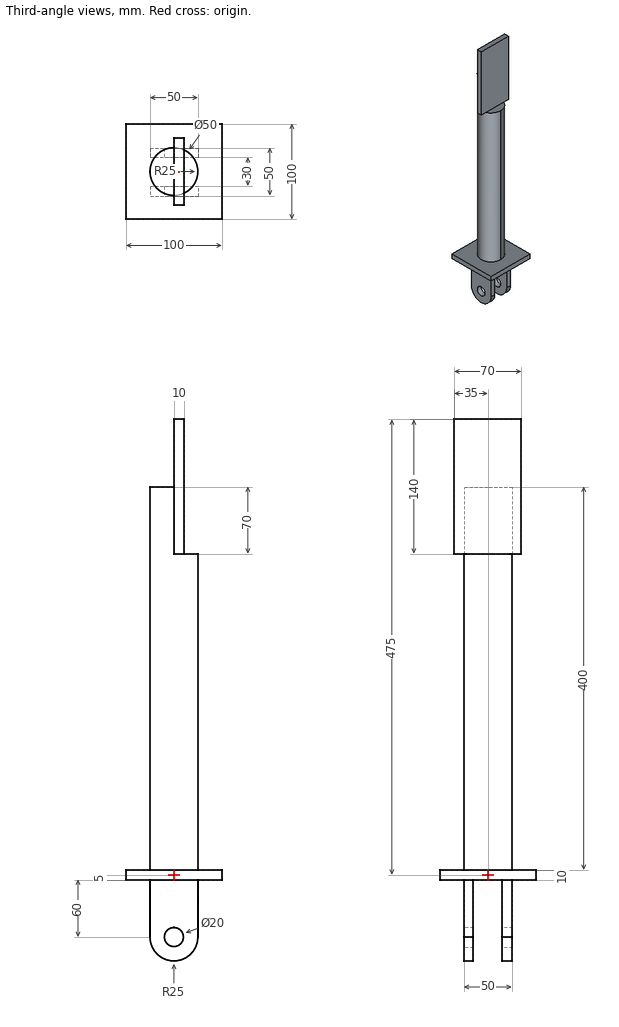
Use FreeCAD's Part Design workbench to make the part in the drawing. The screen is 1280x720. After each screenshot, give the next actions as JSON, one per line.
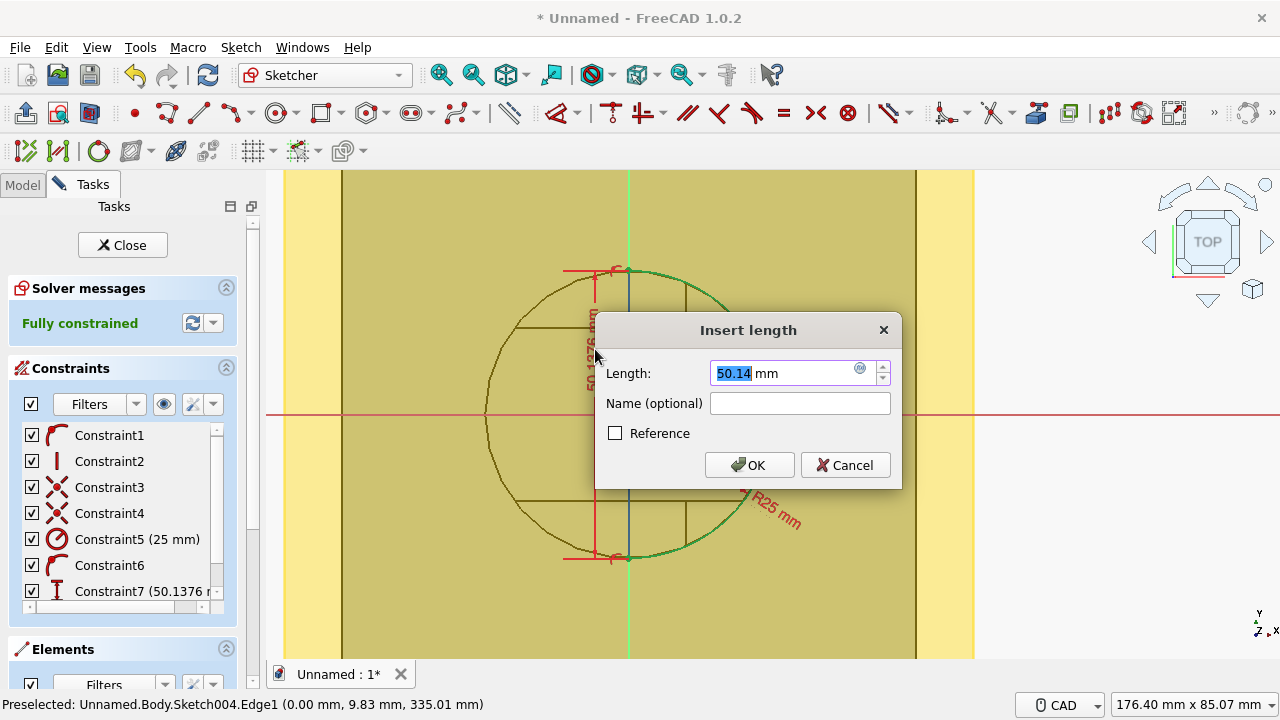
{"action": "type", "text": "50"}
{"action": "key", "text": "Return"}
{"action": "key", "text": "Escape"}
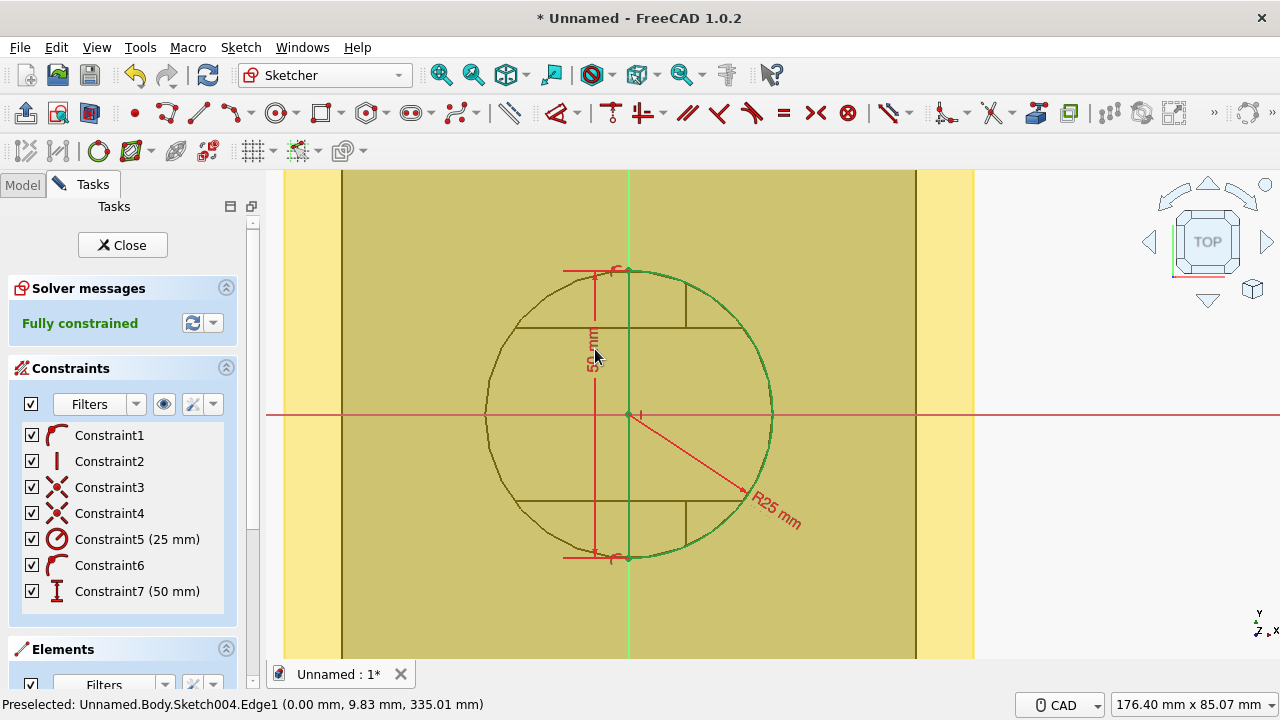
{"action": "left_click", "coordinate": [123, 245]}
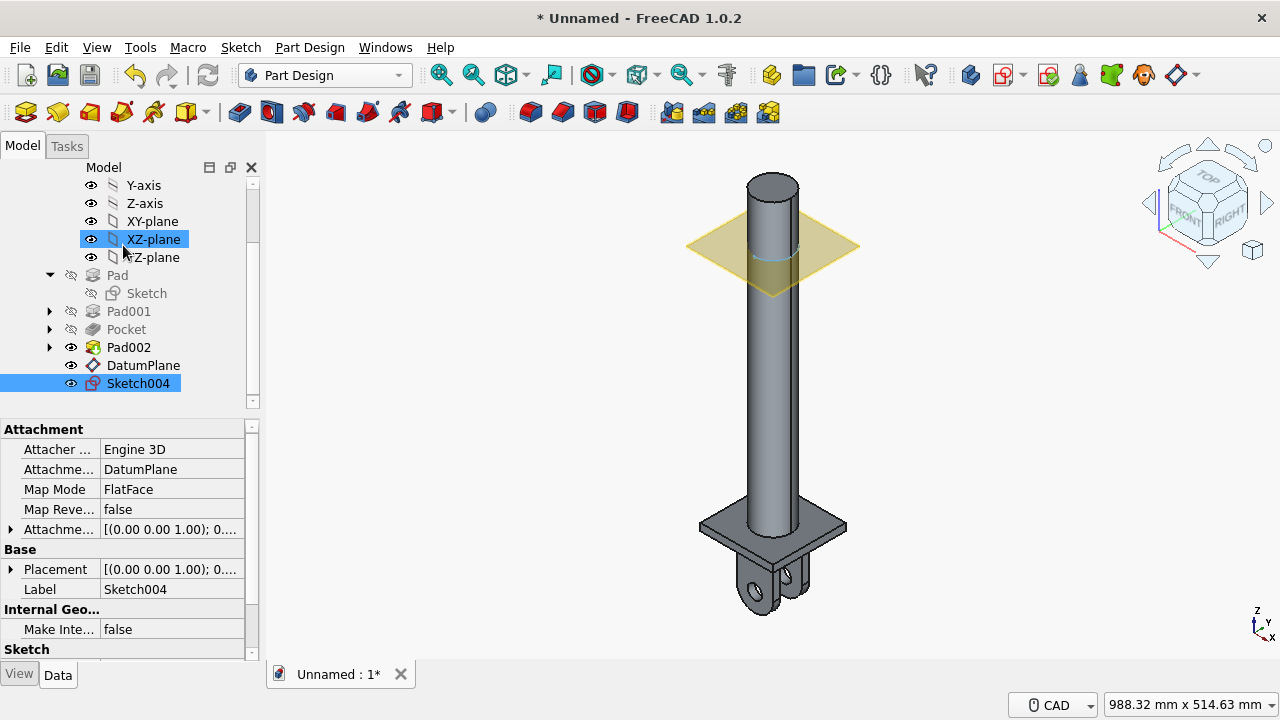
{"action": "left_click", "coordinate": [240, 112]}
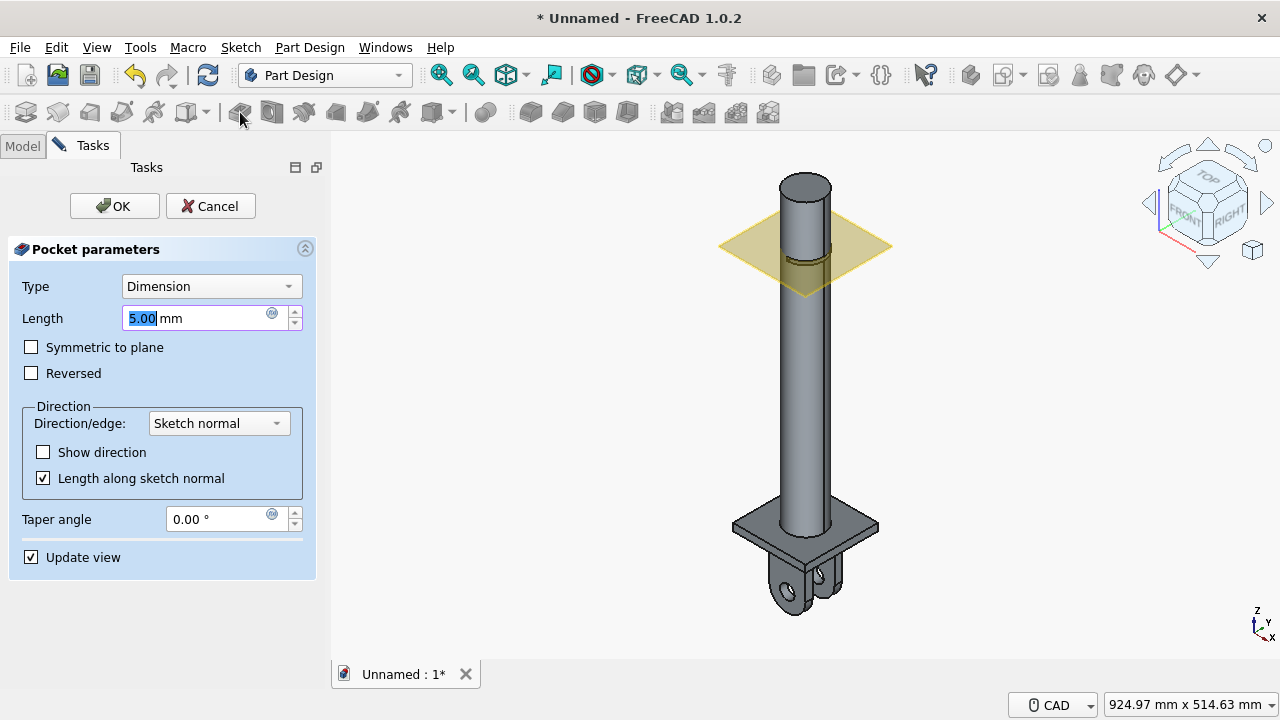
{"action": "type", "text": "70"}
{"action": "key", "text": "Tab"}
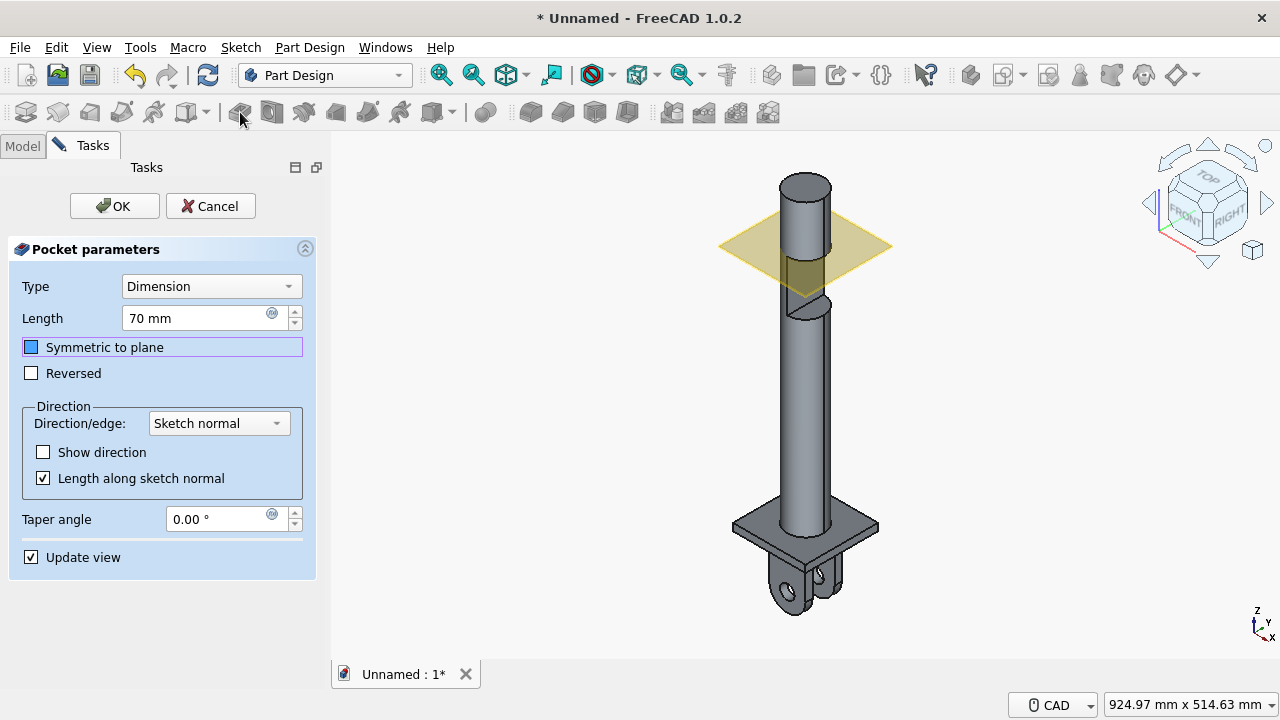
{"action": "left_click", "coordinate": [30, 373]}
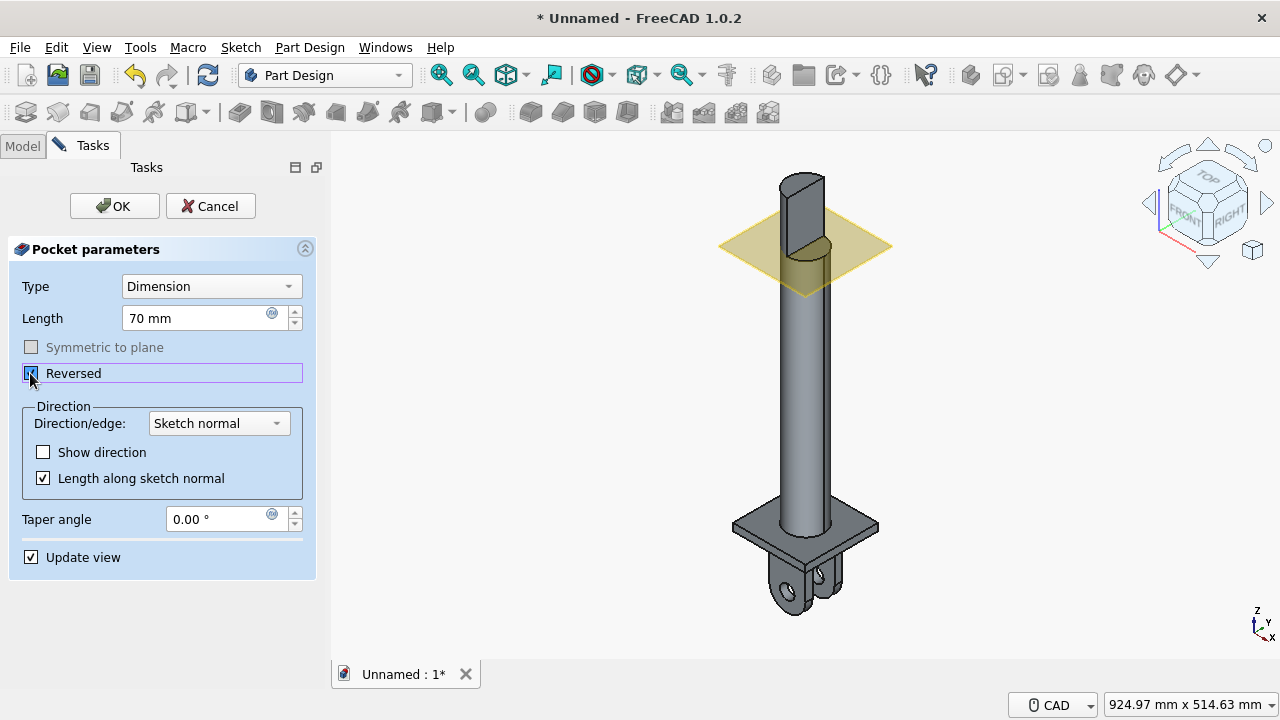
{"action": "left_click", "coordinate": [115, 206]}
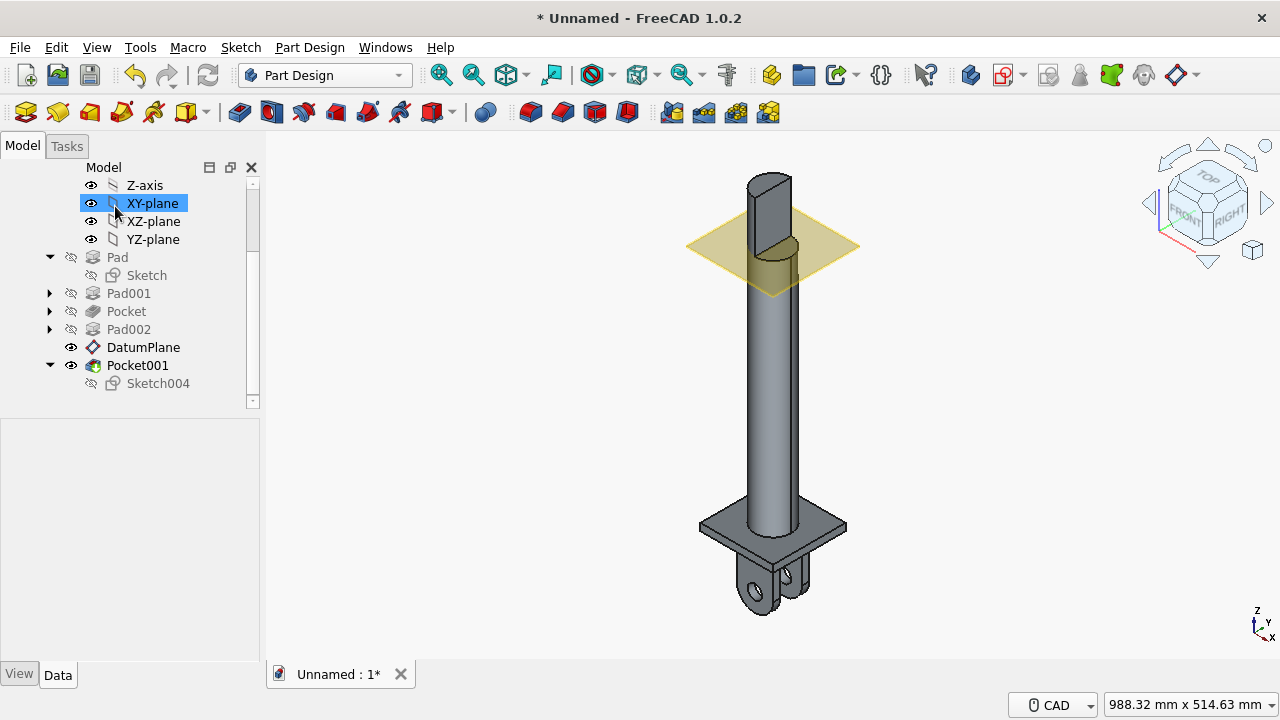
{"action": "left_click", "coordinate": [116, 347]}
{"action": "key", "text": "space"}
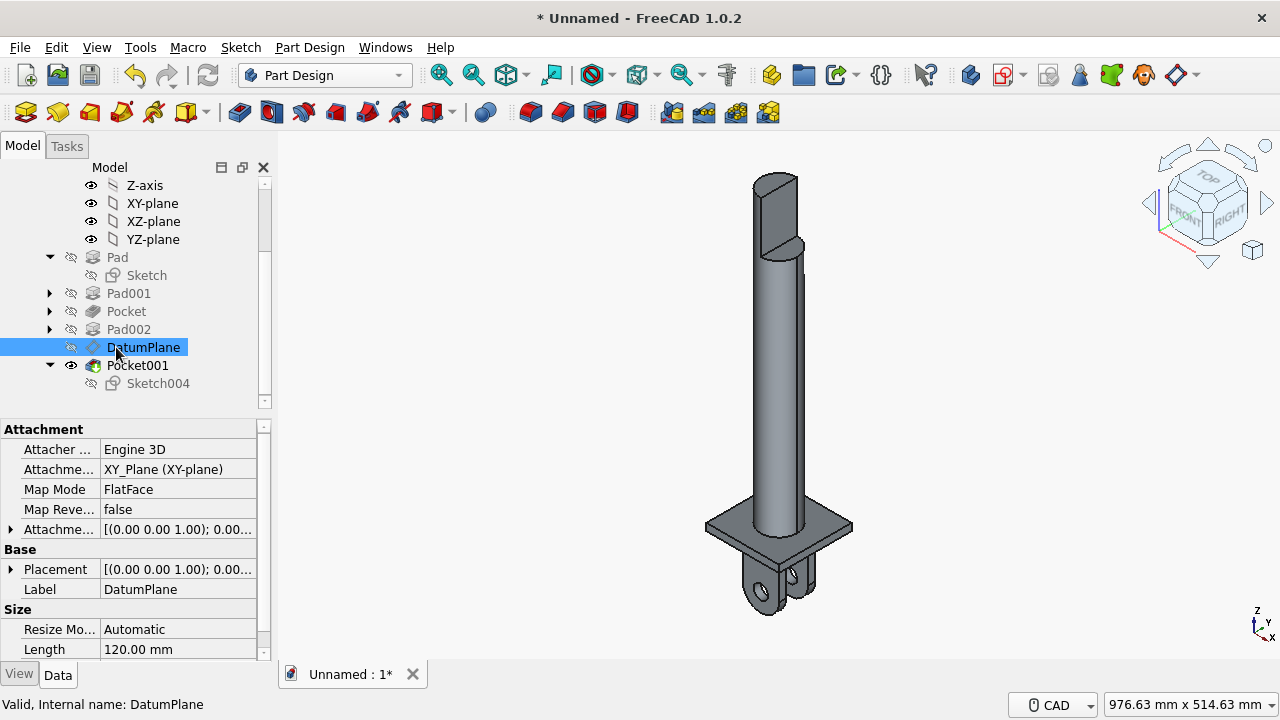
{"action": "left_click", "coordinate": [318, 619]}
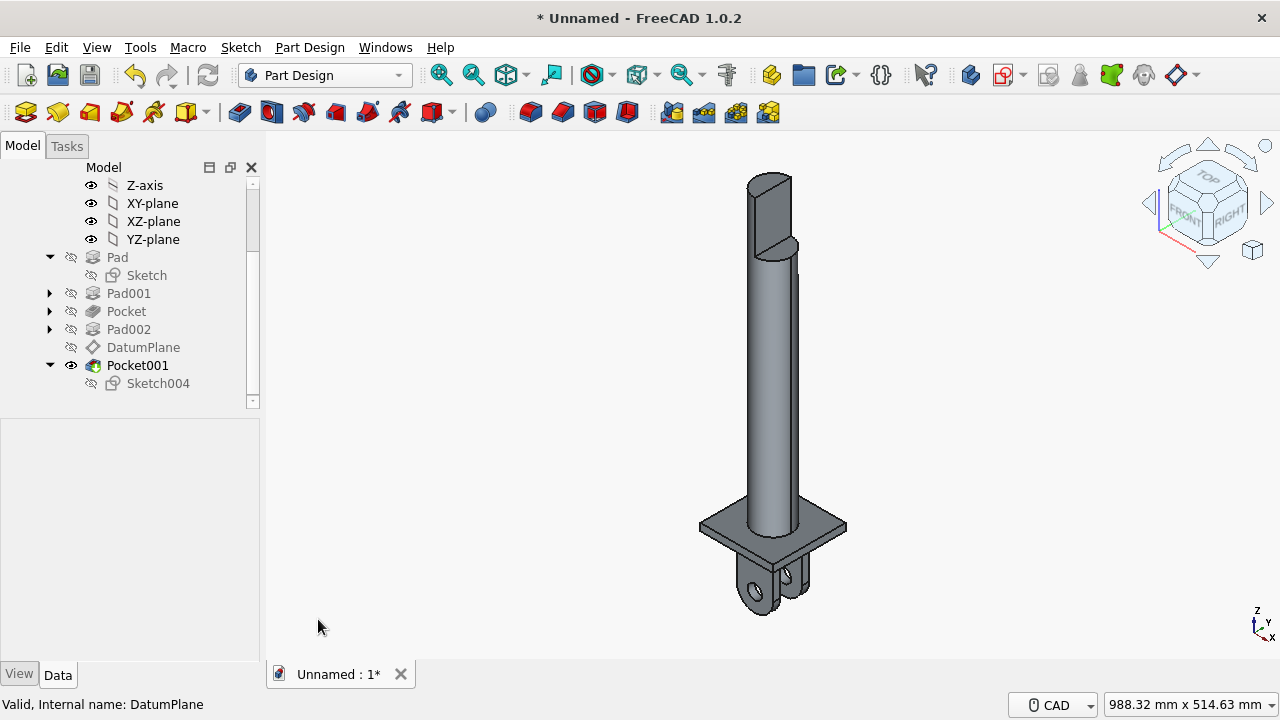
{"action": "left_click", "coordinate": [1004, 76]}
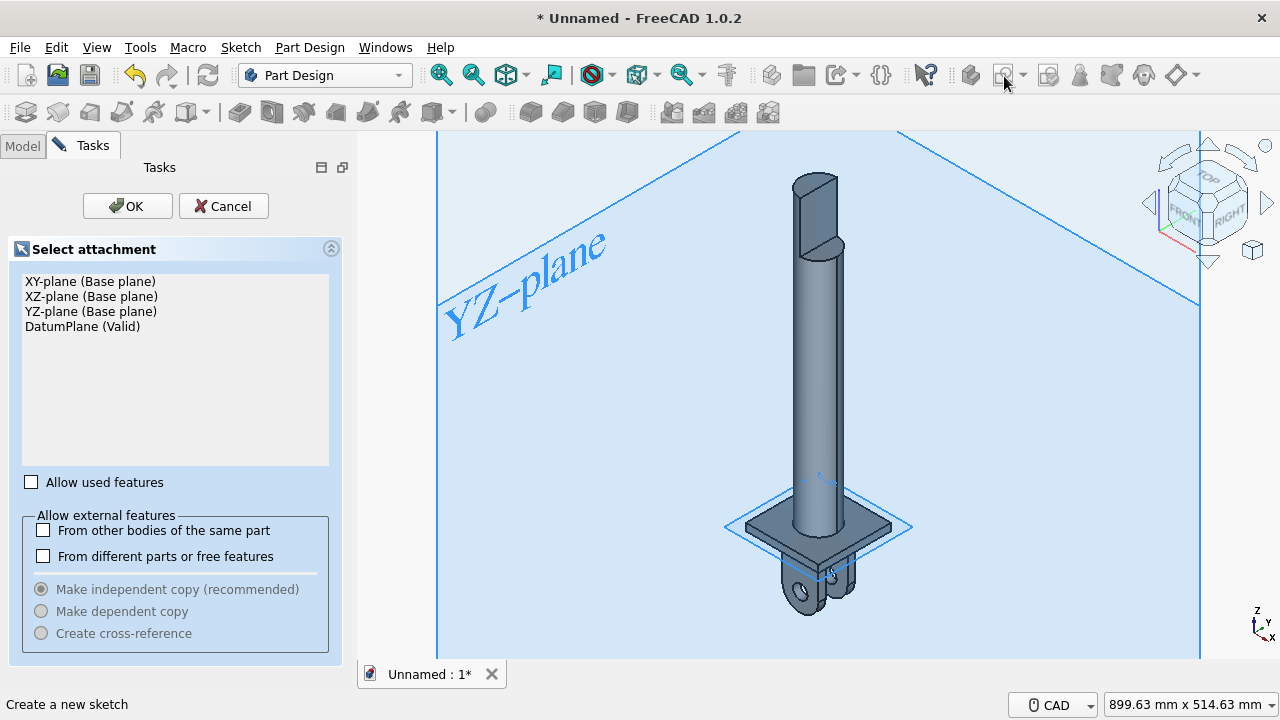
{"action": "left_click", "coordinate": [82, 312]}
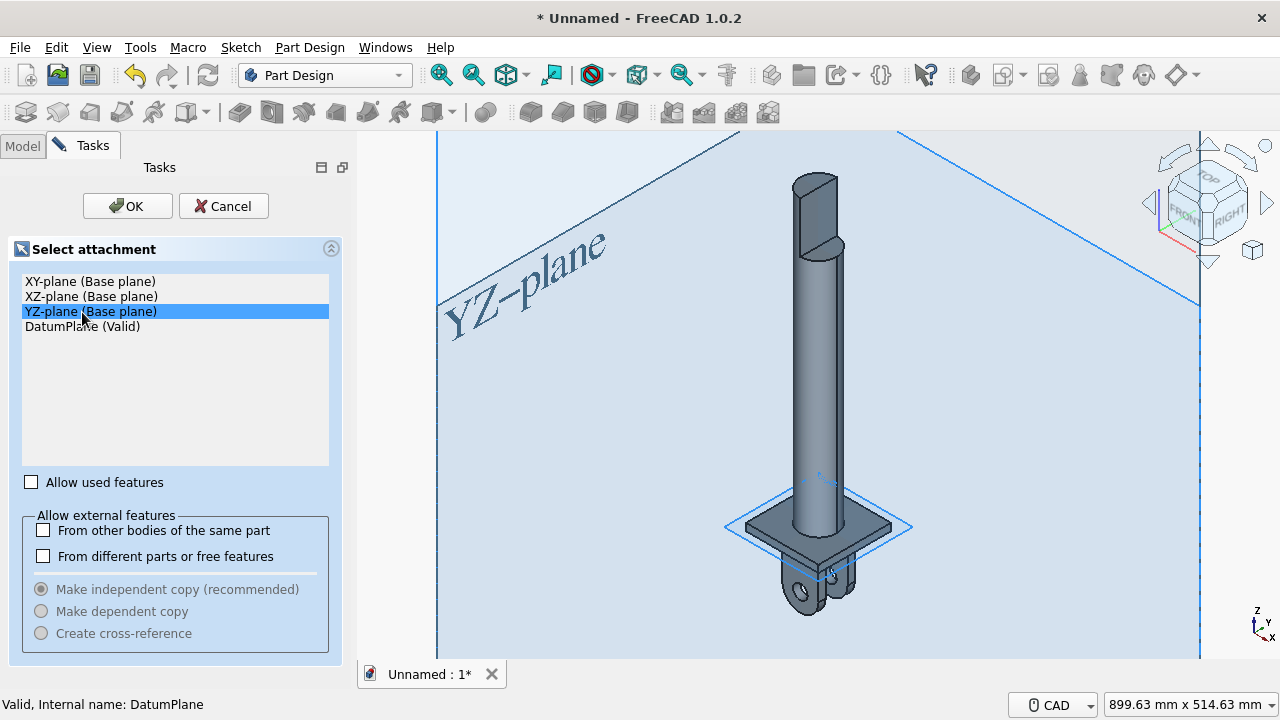
{"action": "left_click", "coordinate": [128, 206]}